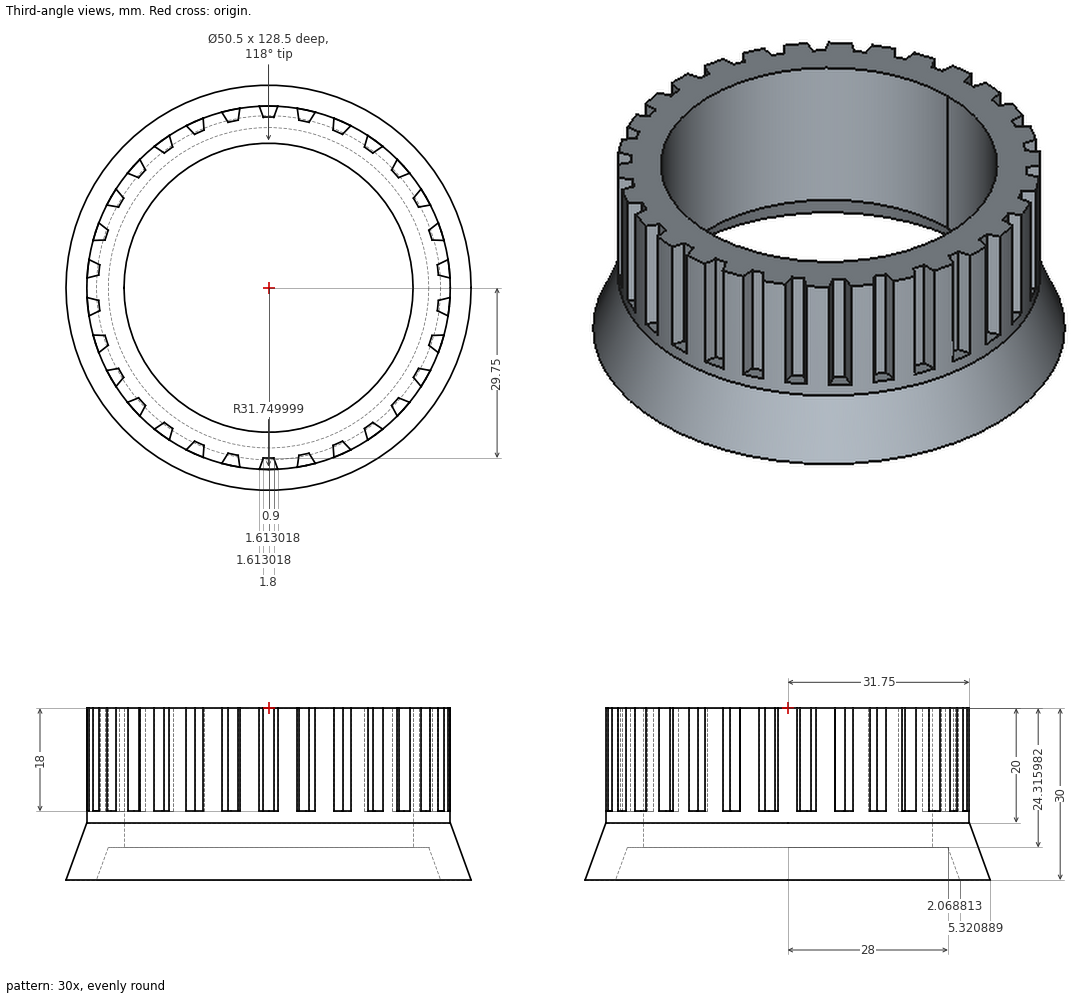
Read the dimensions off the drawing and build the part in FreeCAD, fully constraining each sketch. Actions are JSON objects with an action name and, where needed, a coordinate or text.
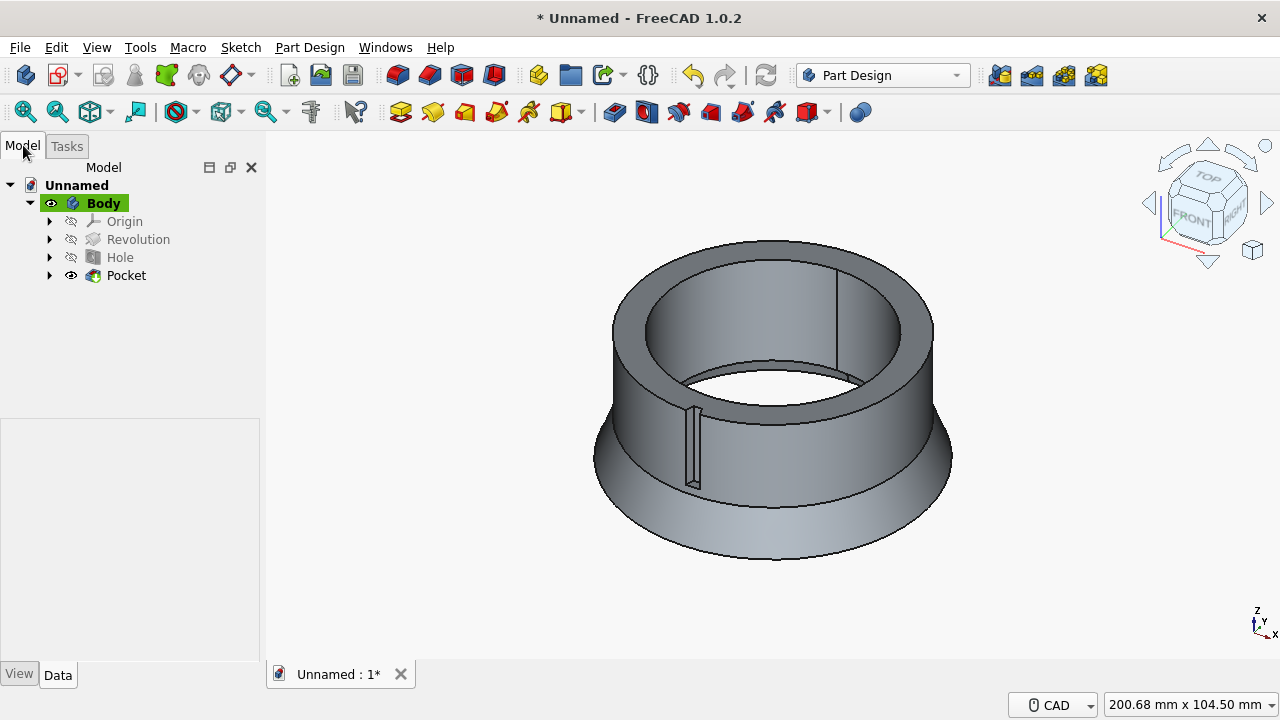
{"action": "left_click", "coordinate": [116, 275]}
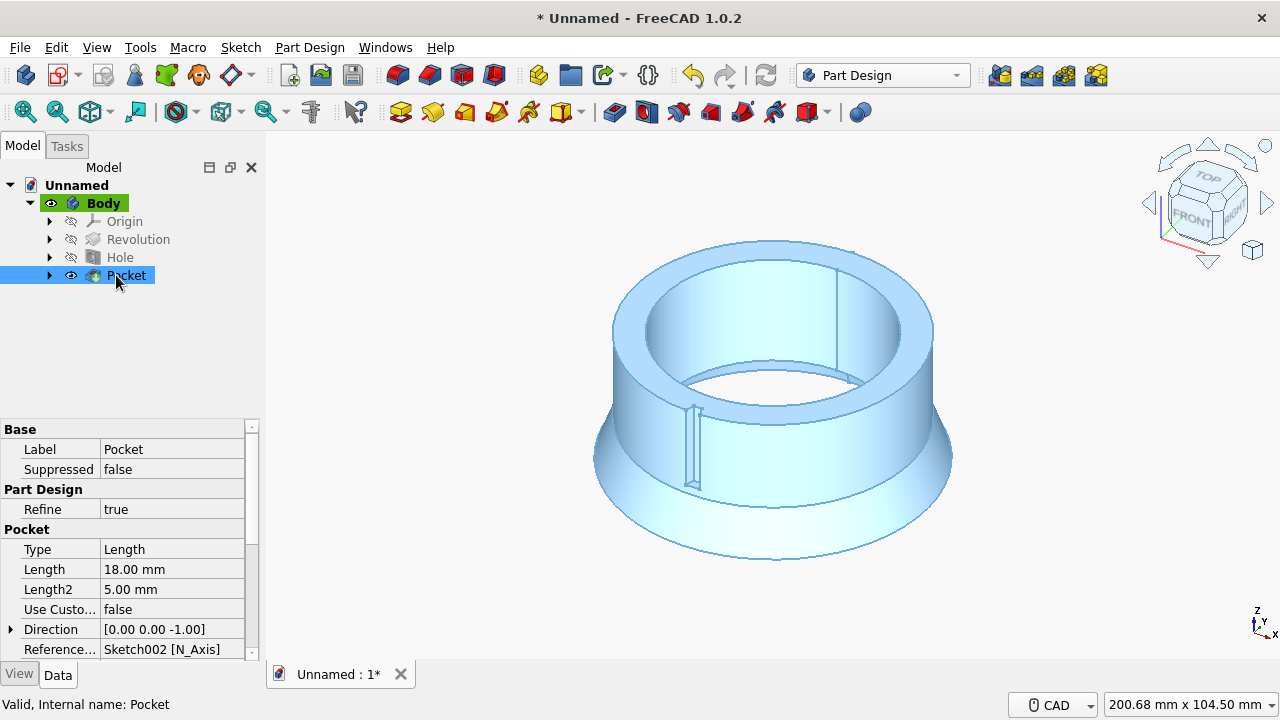
{"action": "left_click", "coordinate": [1064, 76]}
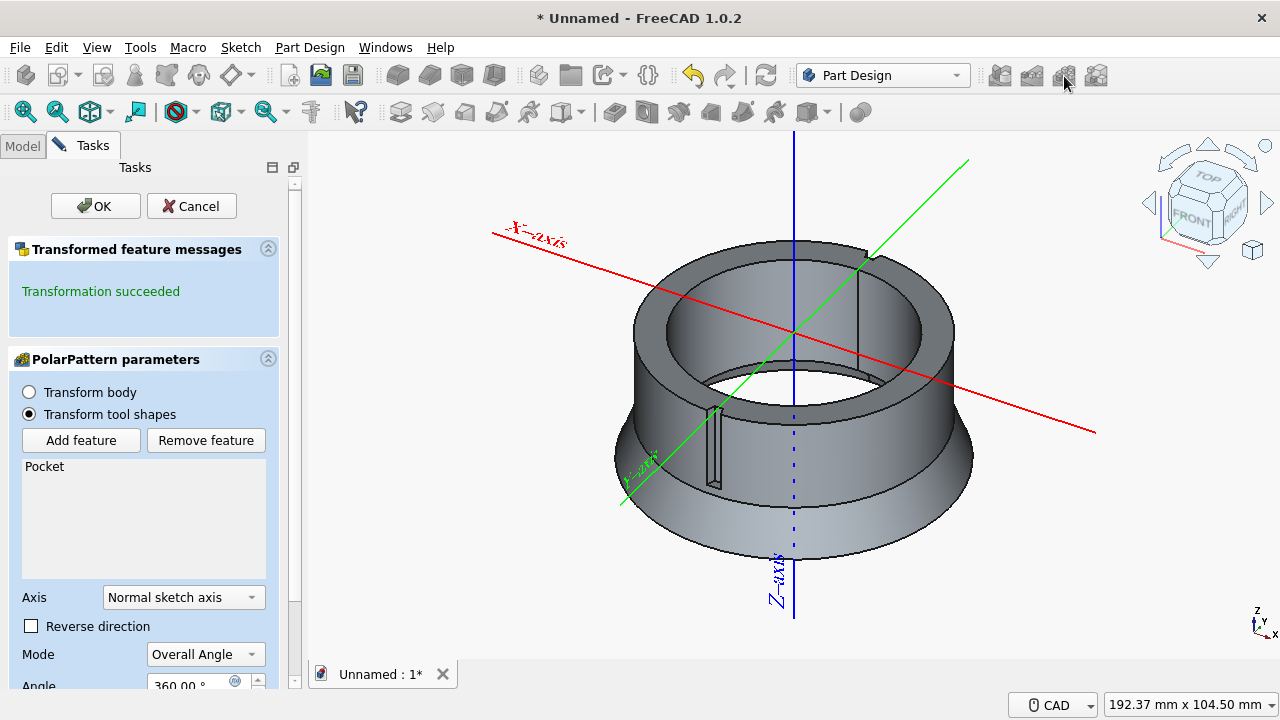
{"action": "left_click", "coordinate": [184, 598]}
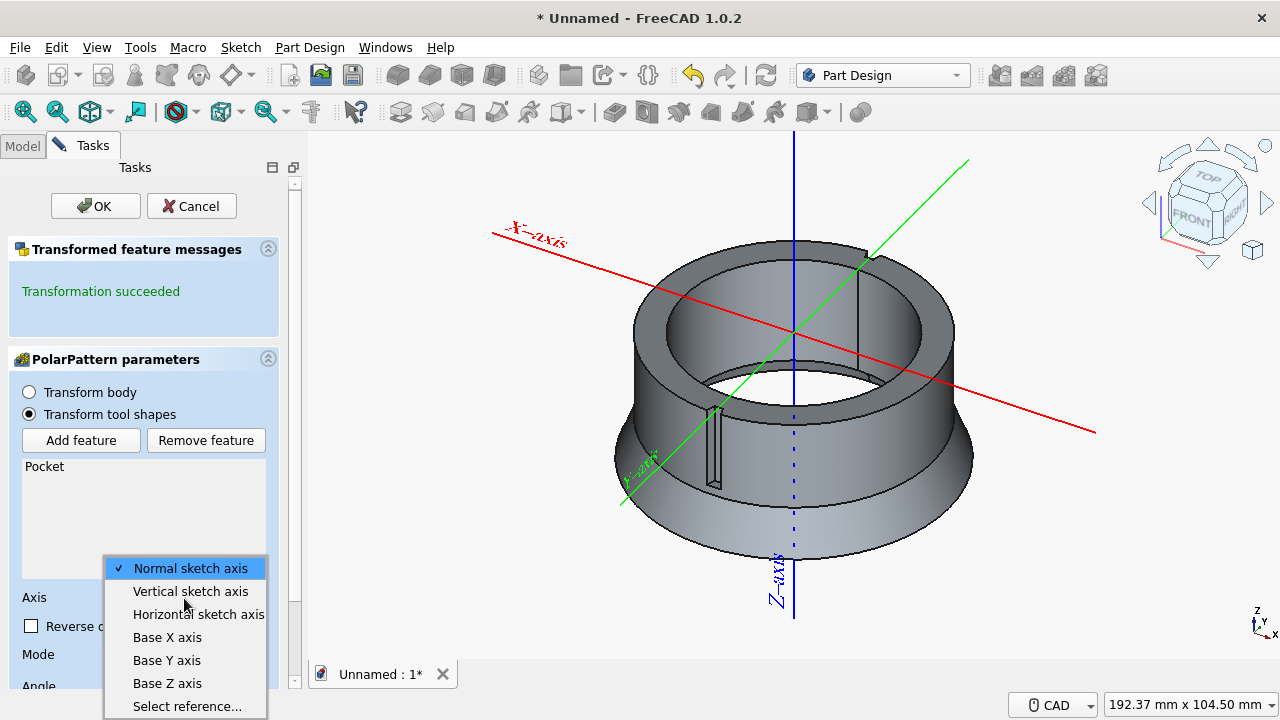
{"action": "left_click", "coordinate": [184, 684]}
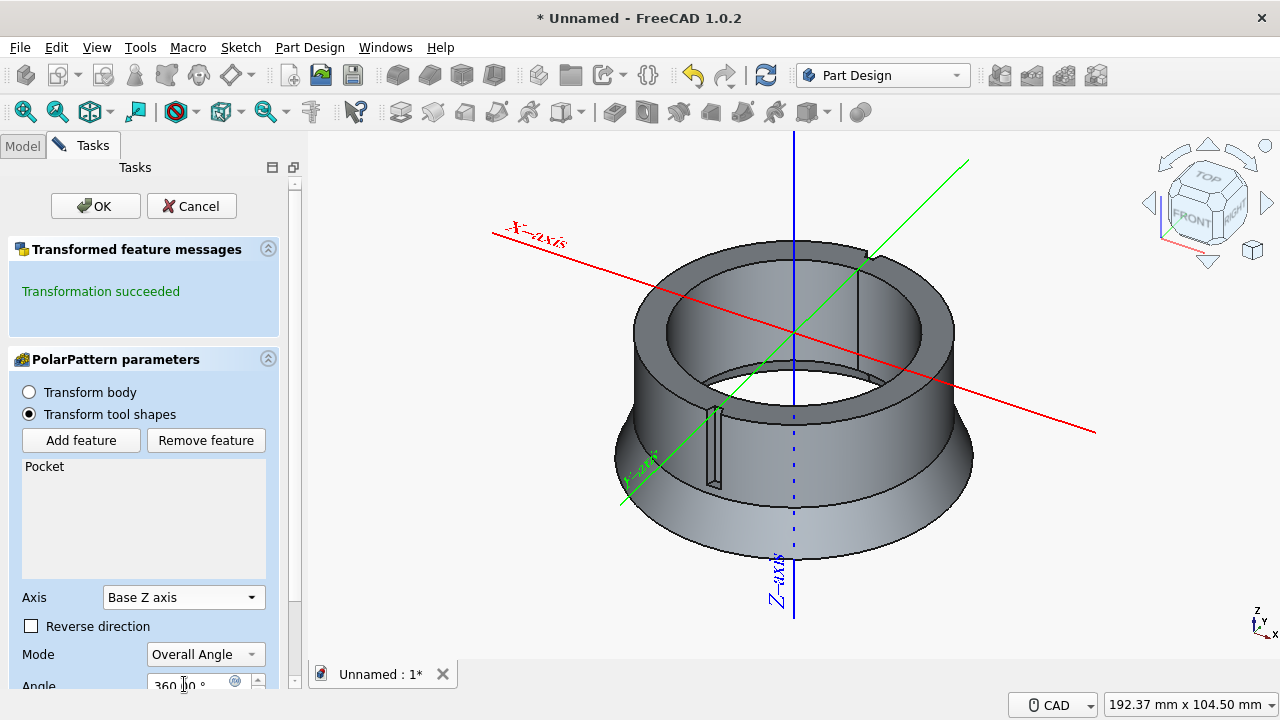
{"action": "scroll", "coordinate": [295, 432], "scroll_direction": "down", "scroll_amount": 2}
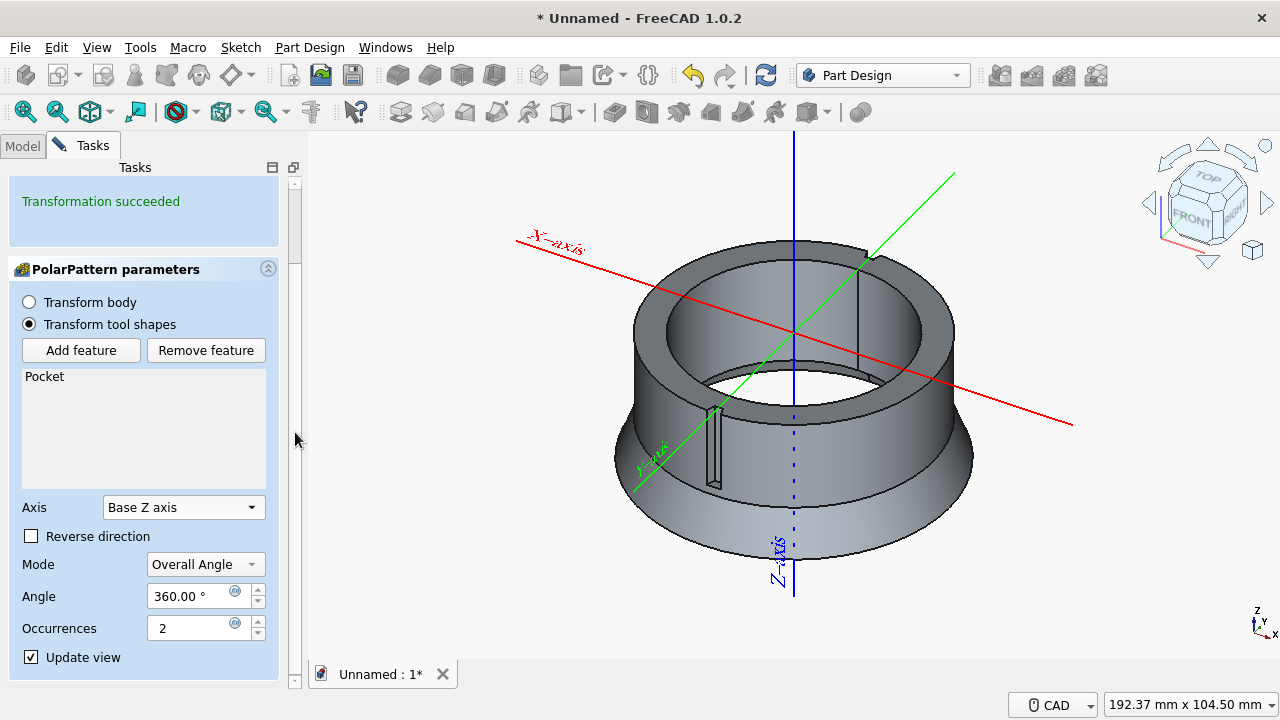
{"action": "triple_click", "coordinate": [198, 628]}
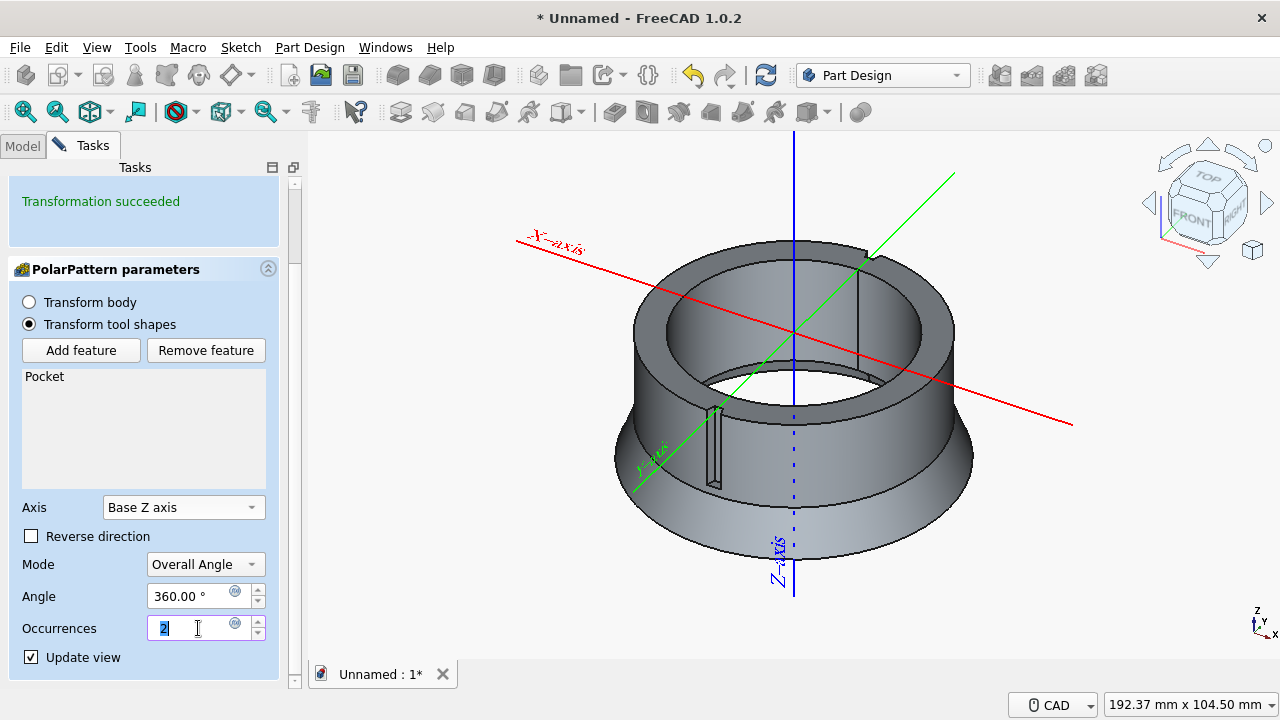
{"action": "type", "text": "30"}
{"action": "key", "text": "Tab"}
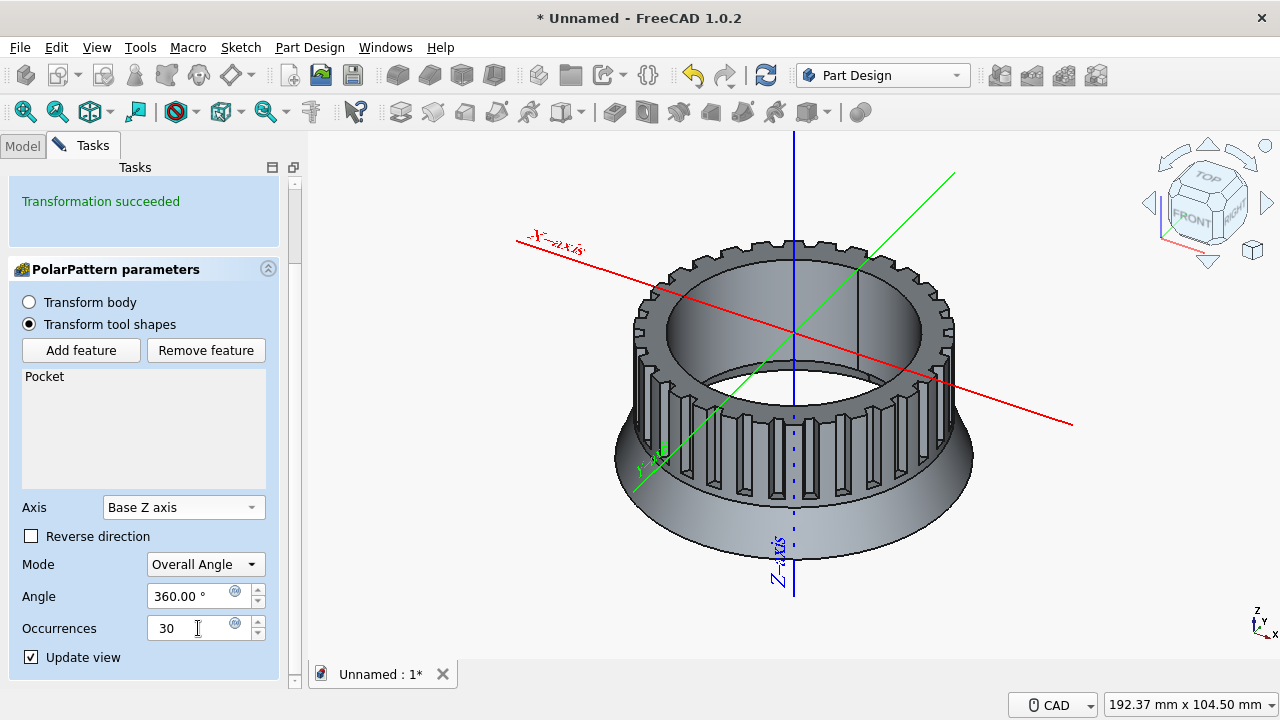
{"action": "scroll", "coordinate": [295, 432], "scroll_direction": "up", "scroll_amount": 3}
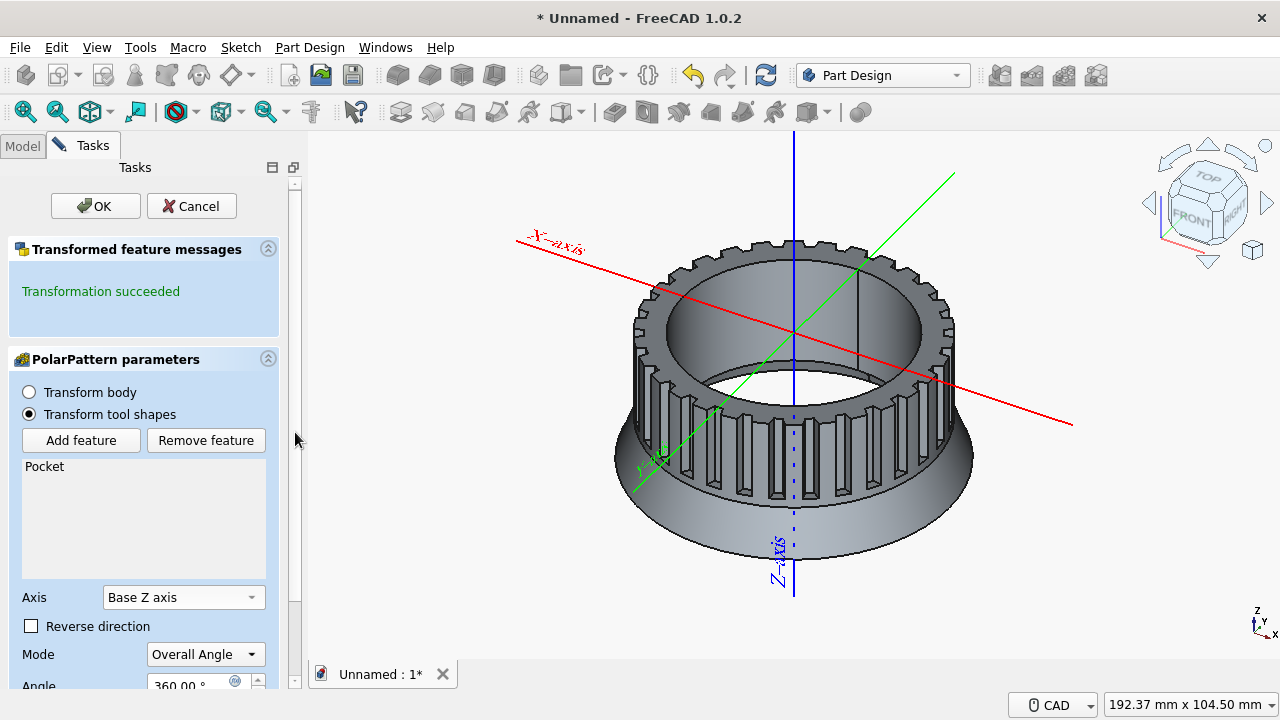
{"action": "left_click", "coordinate": [96, 206]}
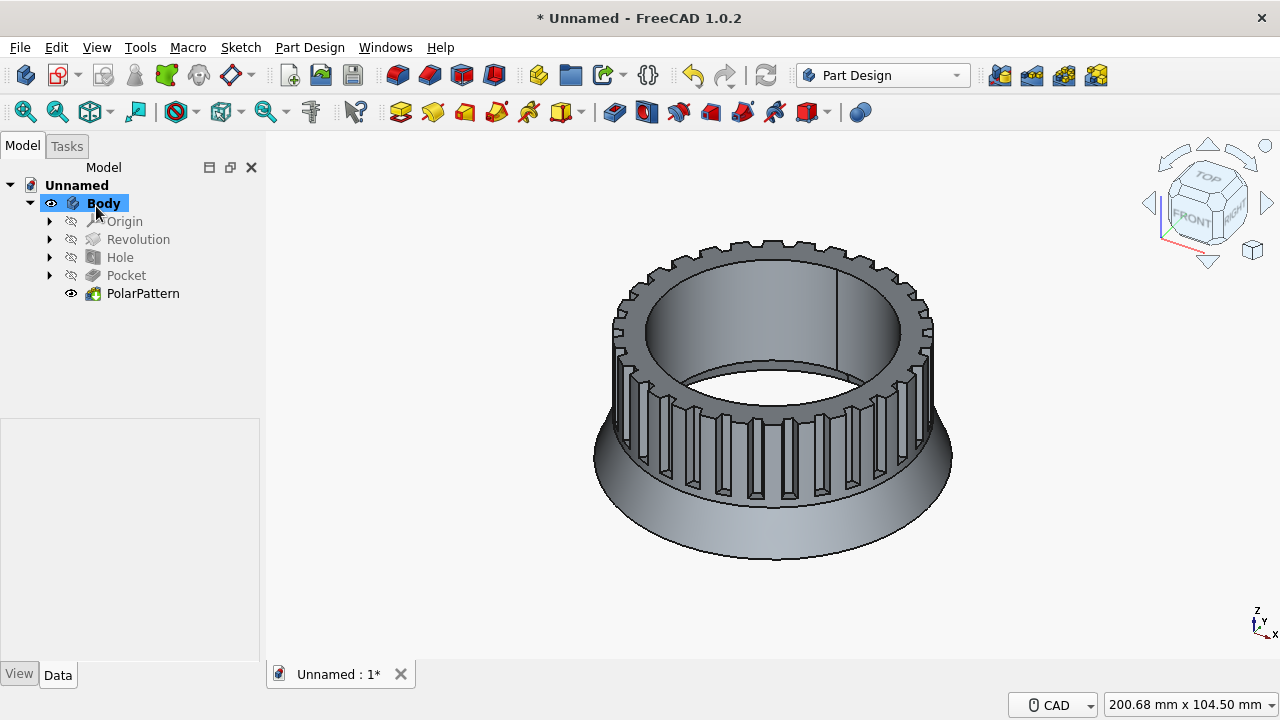
{"action": "key", "text": "0"}